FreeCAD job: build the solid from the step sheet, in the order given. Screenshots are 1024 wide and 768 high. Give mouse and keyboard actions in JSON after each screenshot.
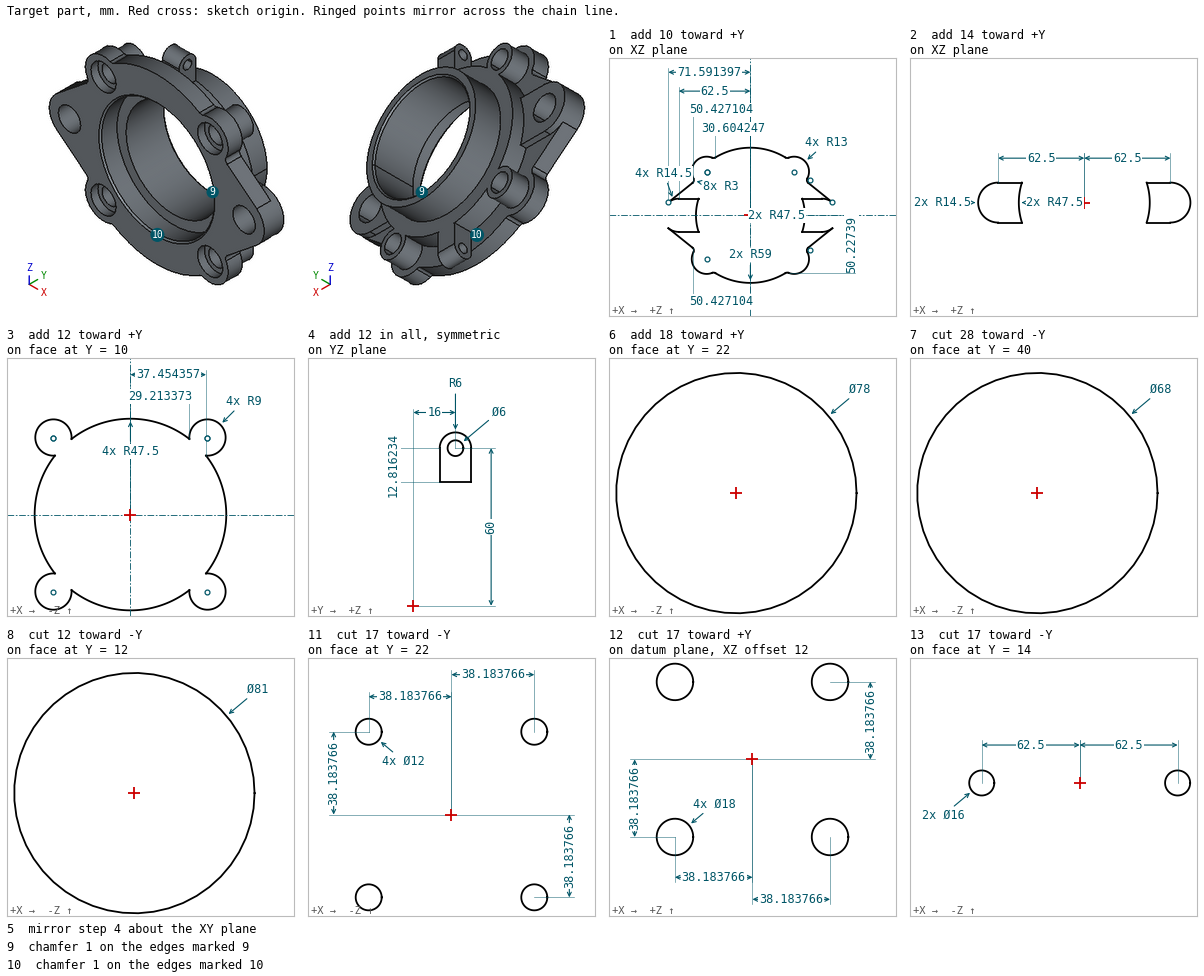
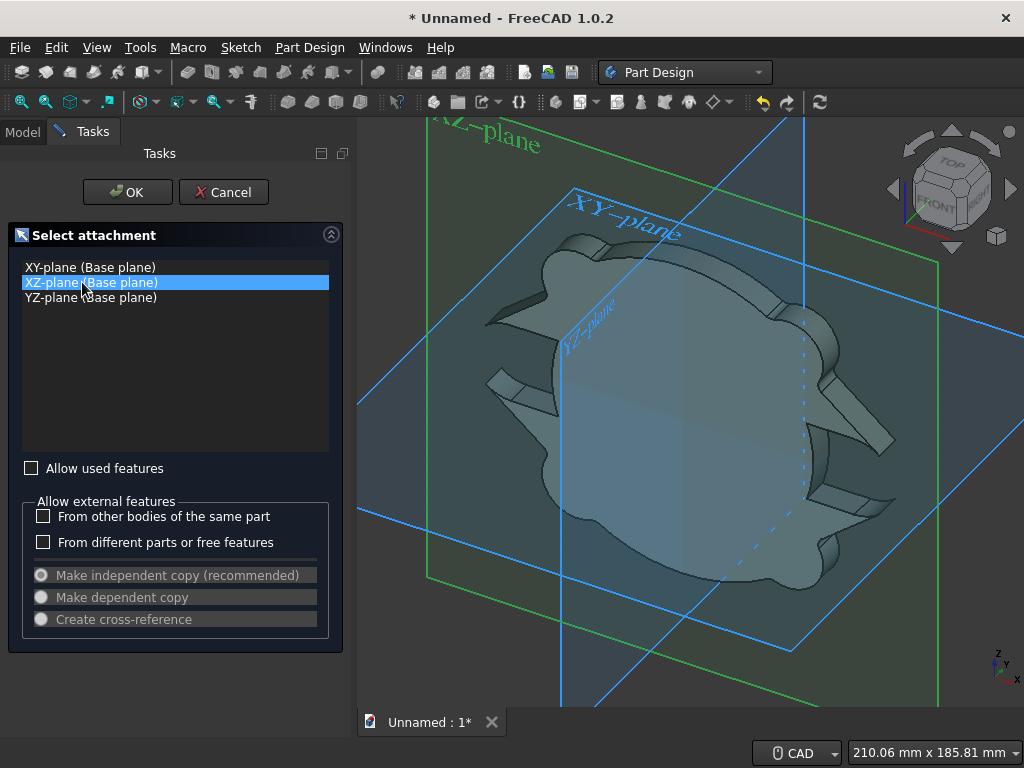
{"action": "left_click", "coordinate": [128, 192]}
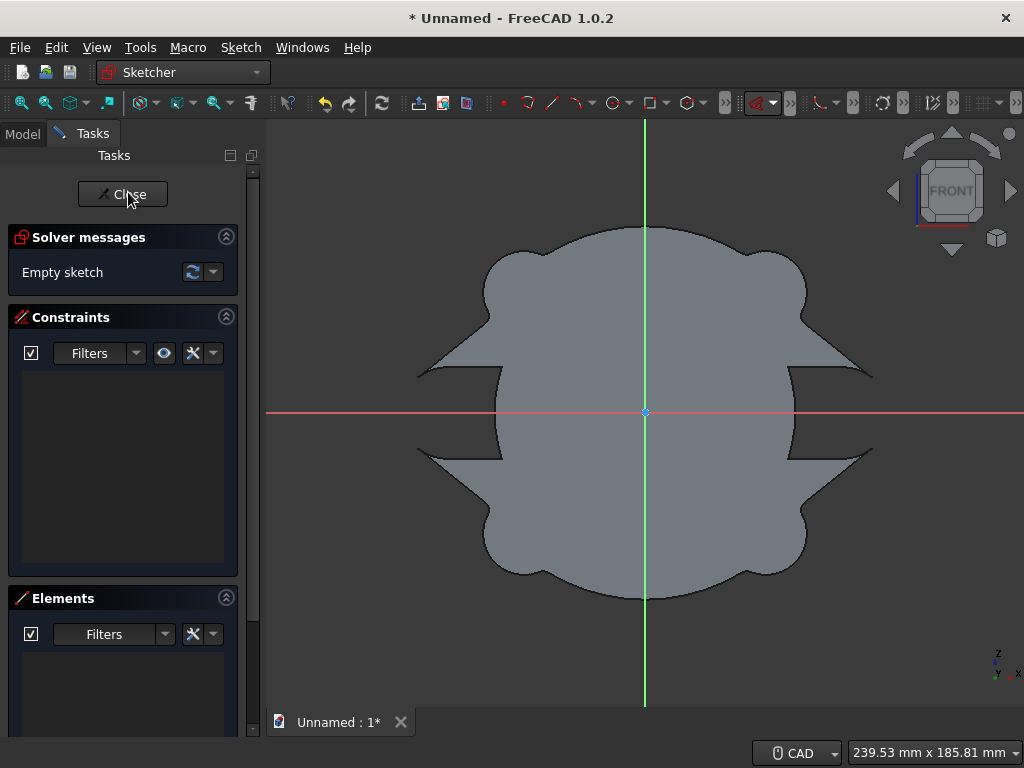
{"action": "scroll", "coordinate": [294, 413], "scroll_direction": "down", "scroll_amount": 1}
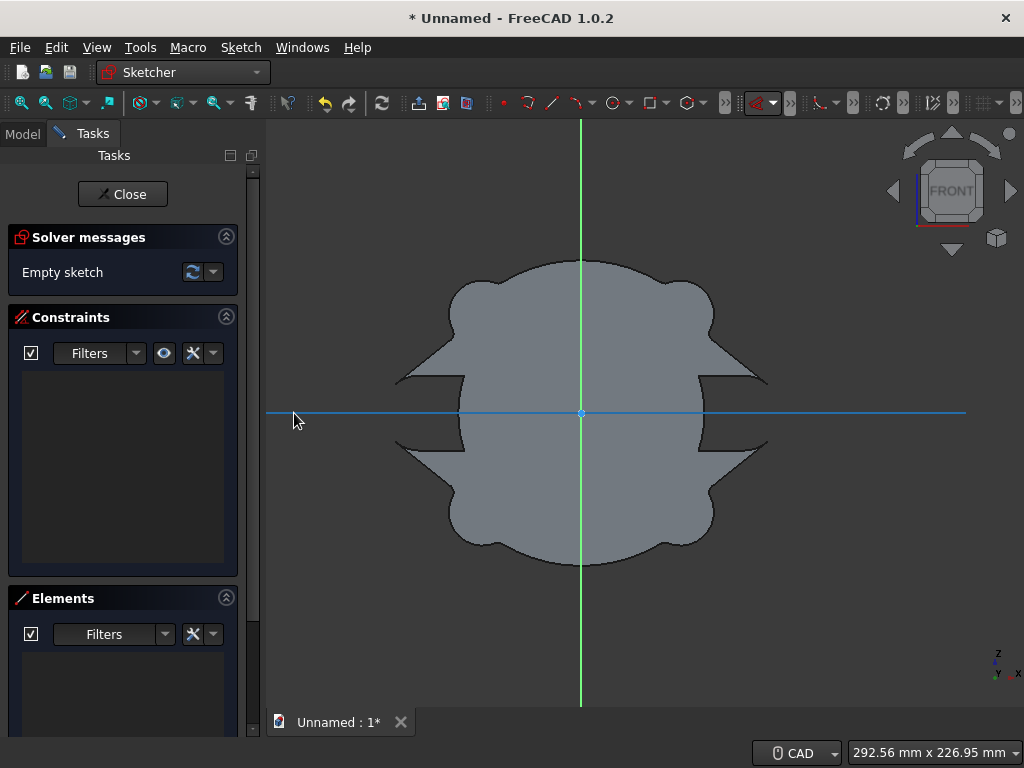
{"action": "key", "text": "g l"}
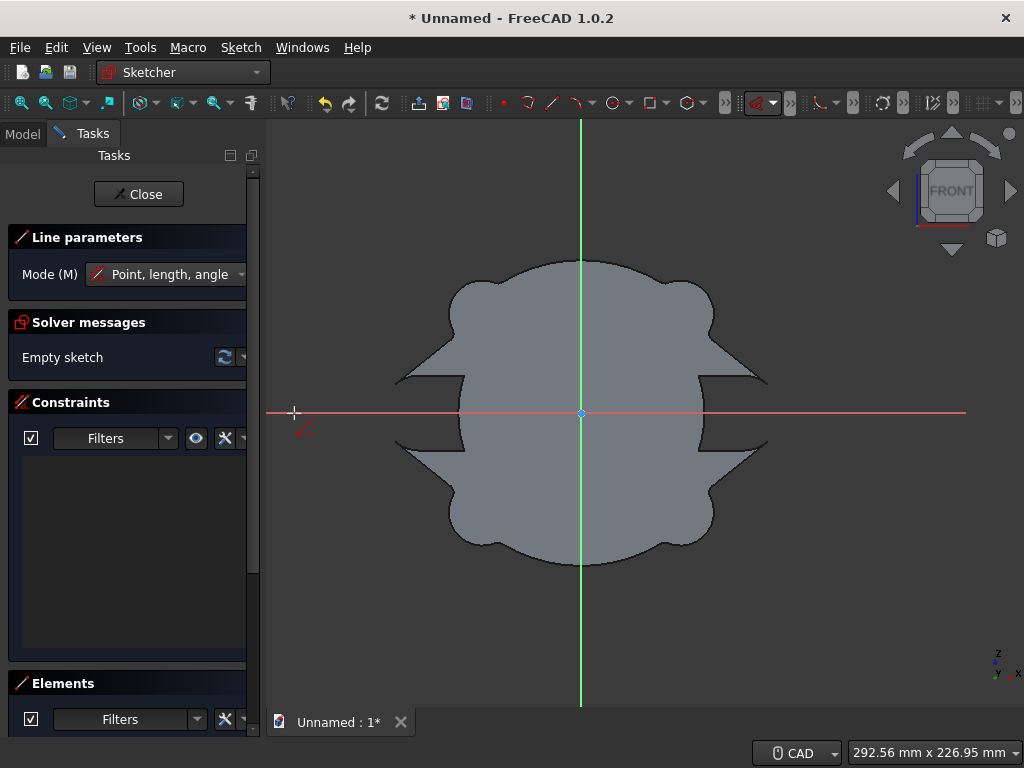
{"action": "left_click", "coordinate": [419, 376]}
{"action": "left_click", "coordinate": [464, 376]}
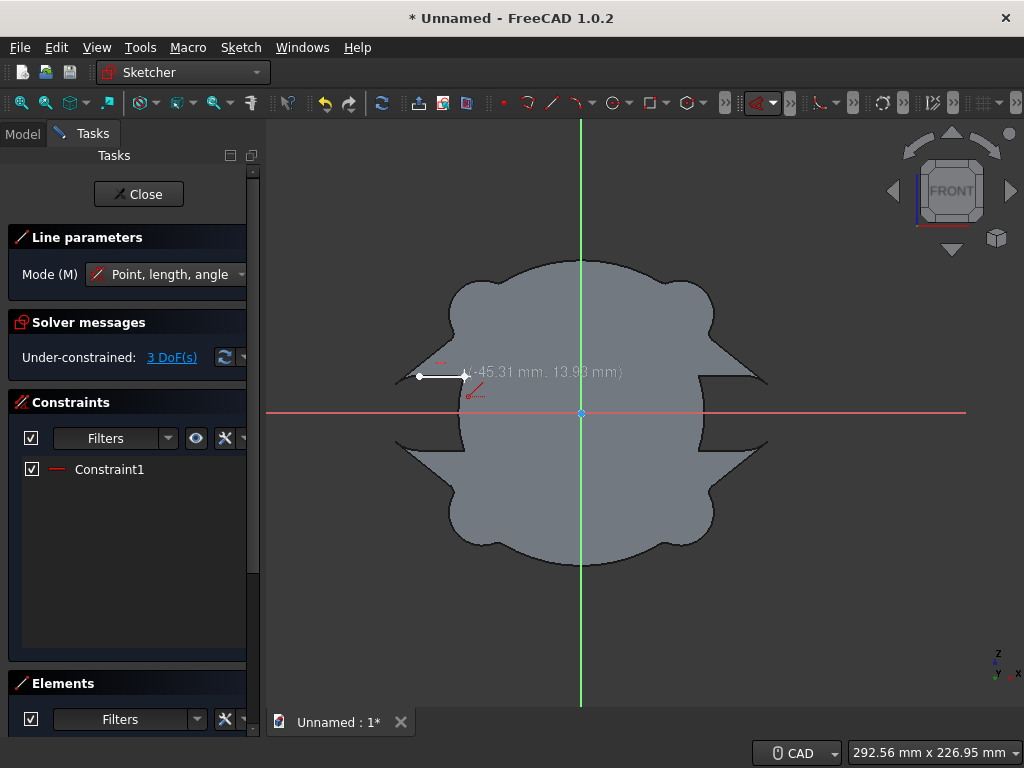
{"action": "left_click", "coordinate": [464, 451]}
{"action": "left_click", "coordinate": [419, 451]}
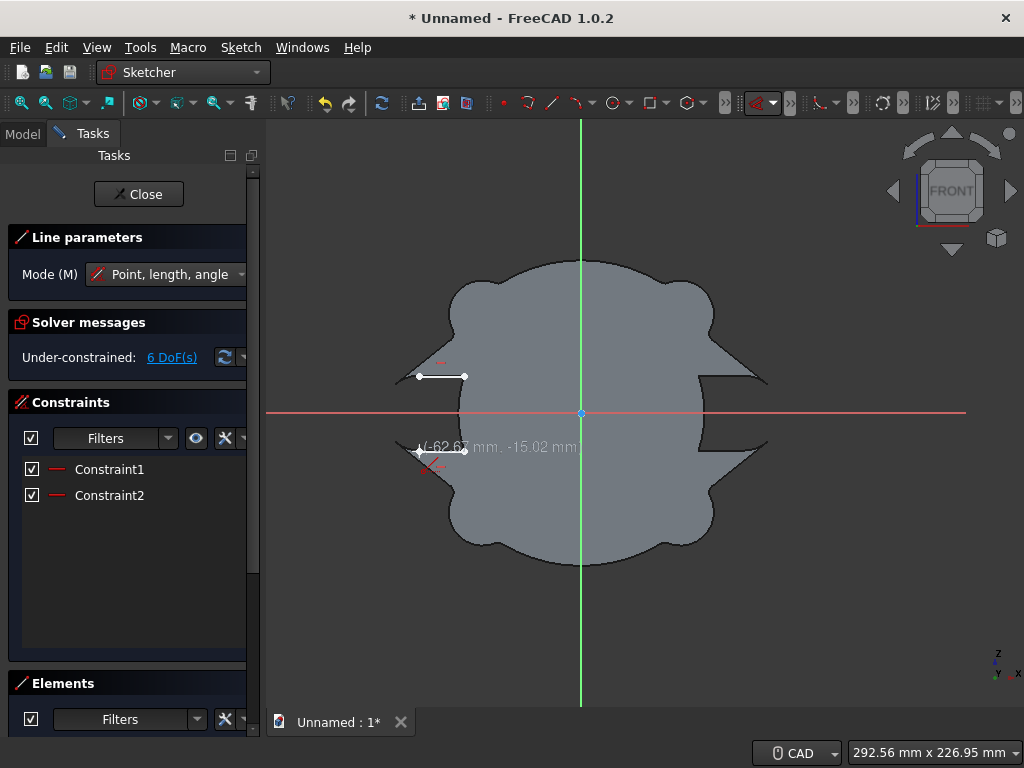
{"action": "key", "text": "g 3 a"}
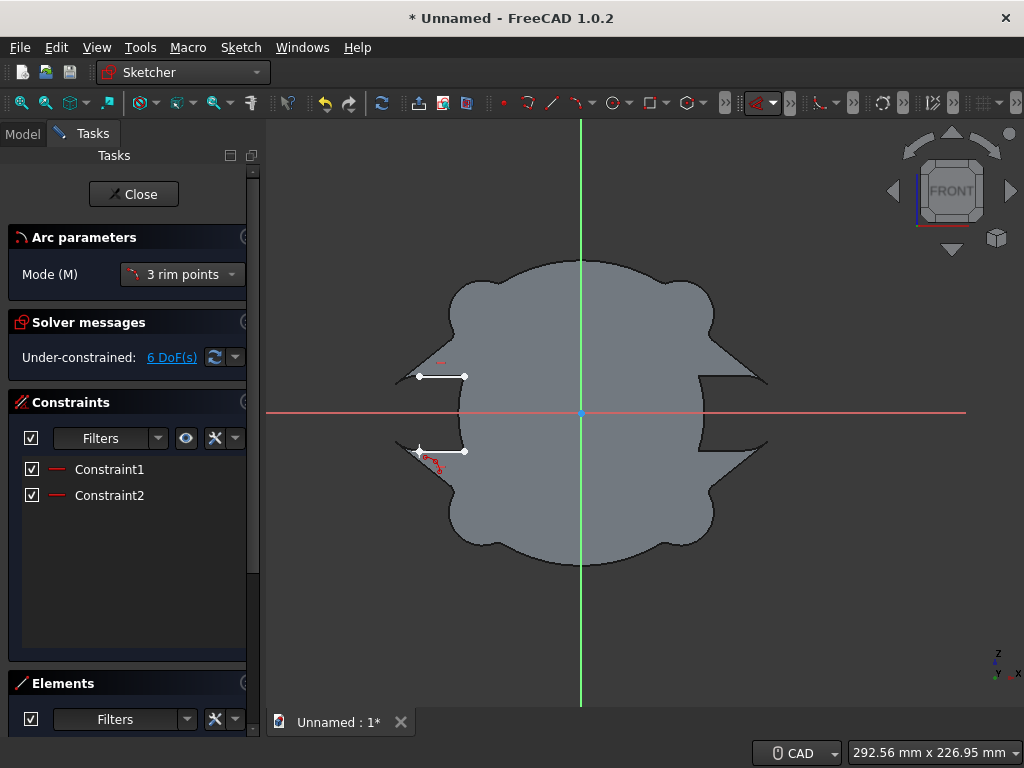
{"action": "left_click", "coordinate": [464, 377]}
{"action": "left_click", "coordinate": [464, 452]}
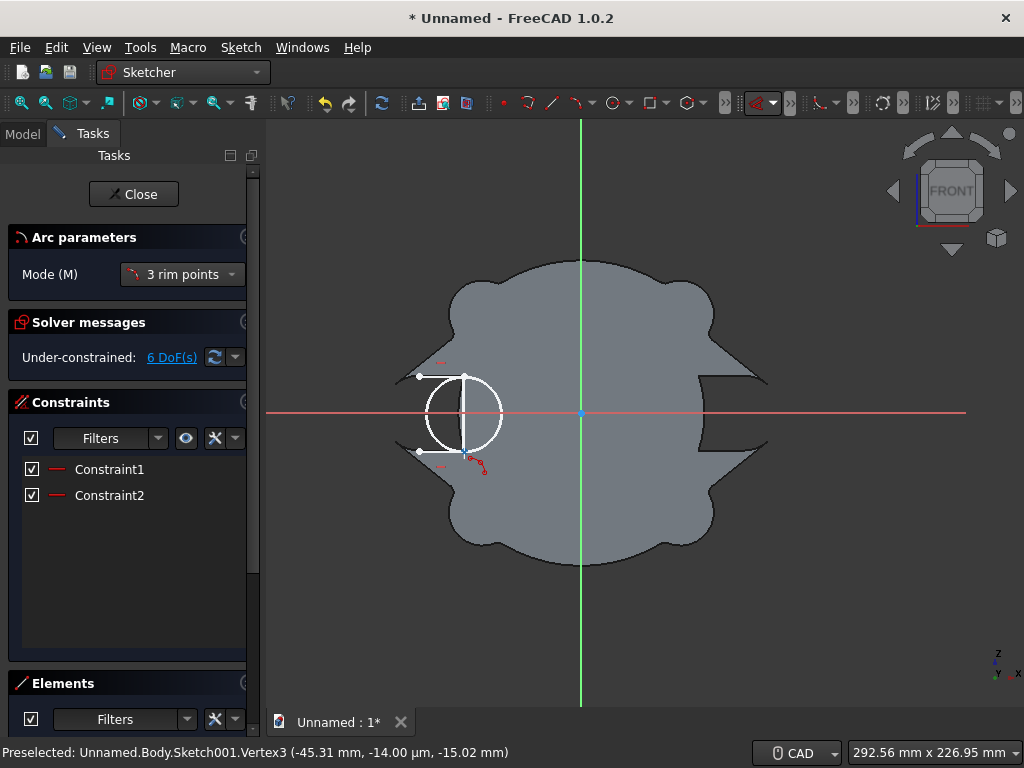
{"action": "scroll", "coordinate": [459, 421], "scroll_direction": "up", "scroll_amount": 6}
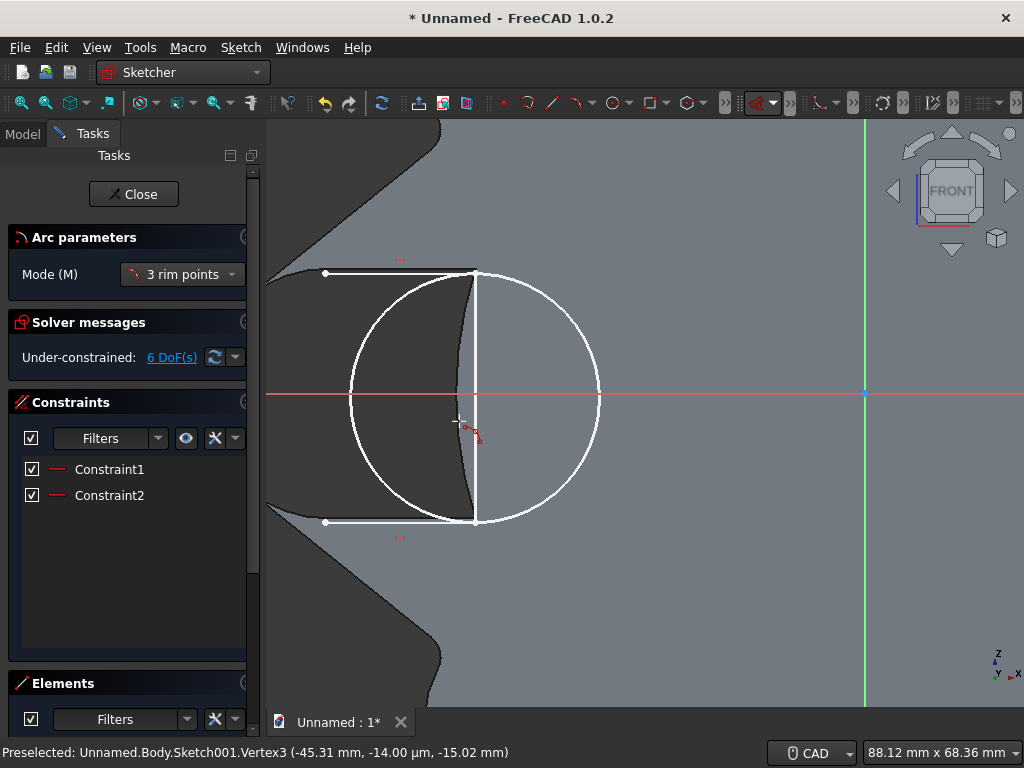
{"action": "left_click", "coordinate": [457, 419]}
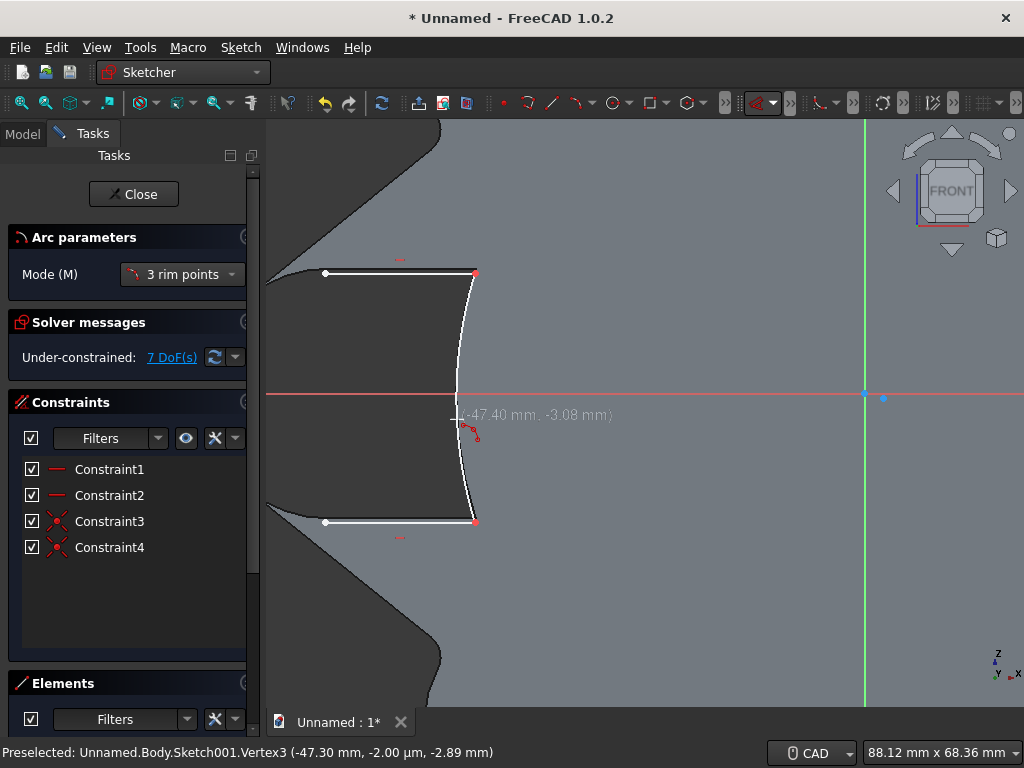
{"action": "left_click", "coordinate": [326, 523]}
{"action": "left_click", "coordinate": [326, 274]}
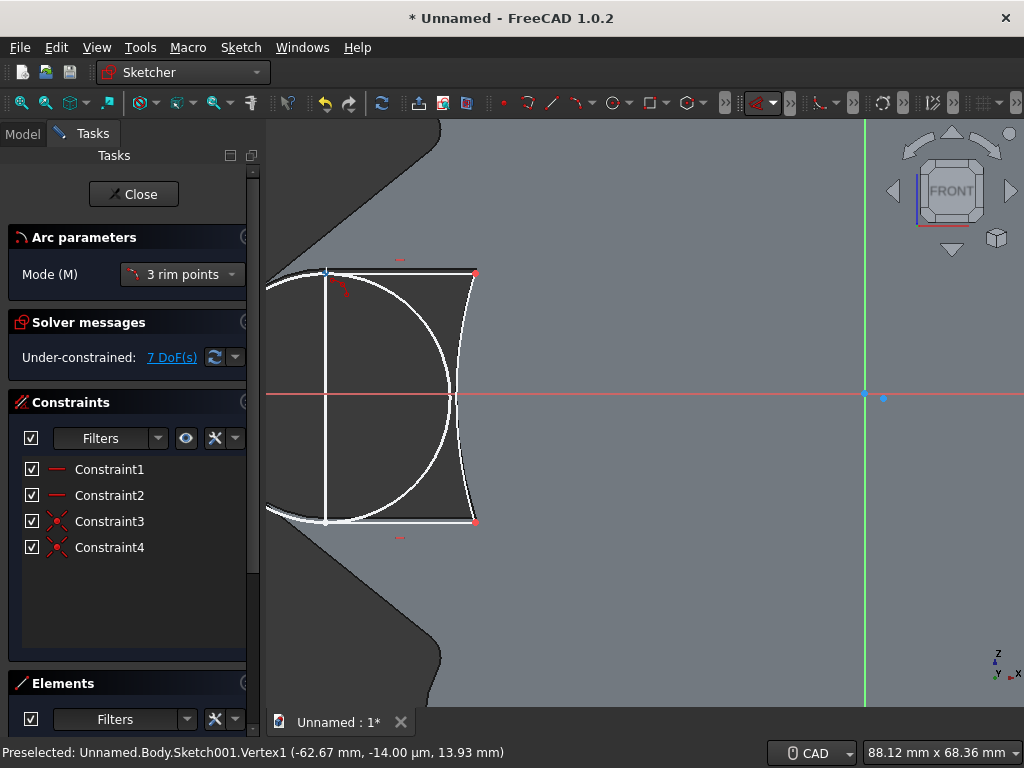
{"action": "scroll", "coordinate": [452, 421], "scroll_direction": "down", "scroll_amount": 6}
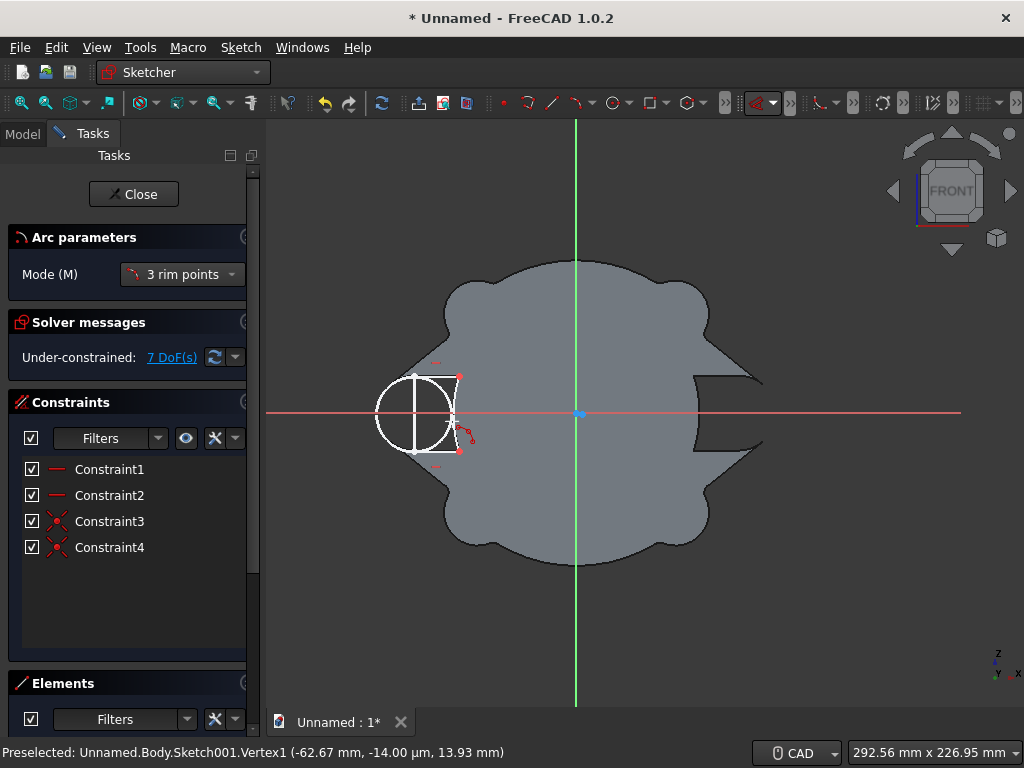
{"action": "left_click", "coordinate": [384, 391]}